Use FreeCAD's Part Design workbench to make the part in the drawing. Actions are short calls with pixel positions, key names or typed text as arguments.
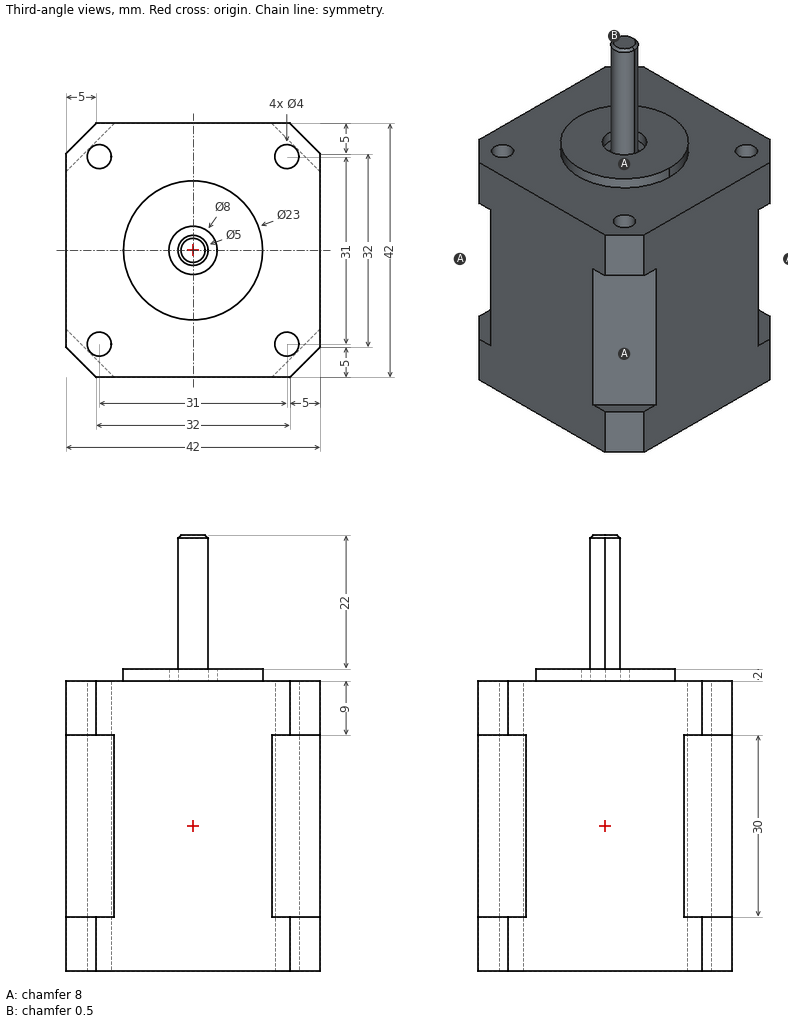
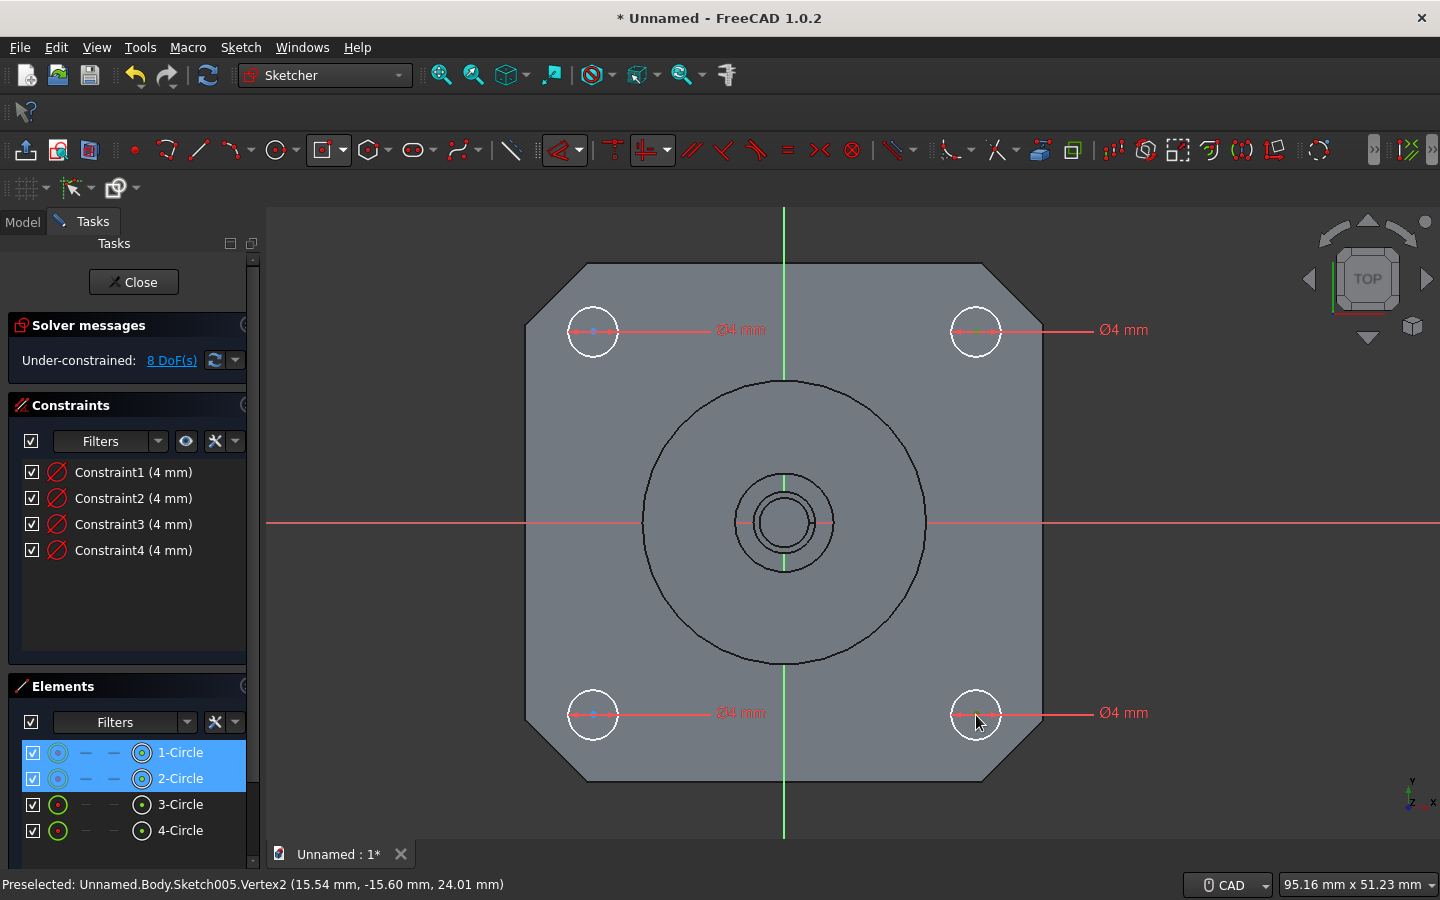
click(364, 523)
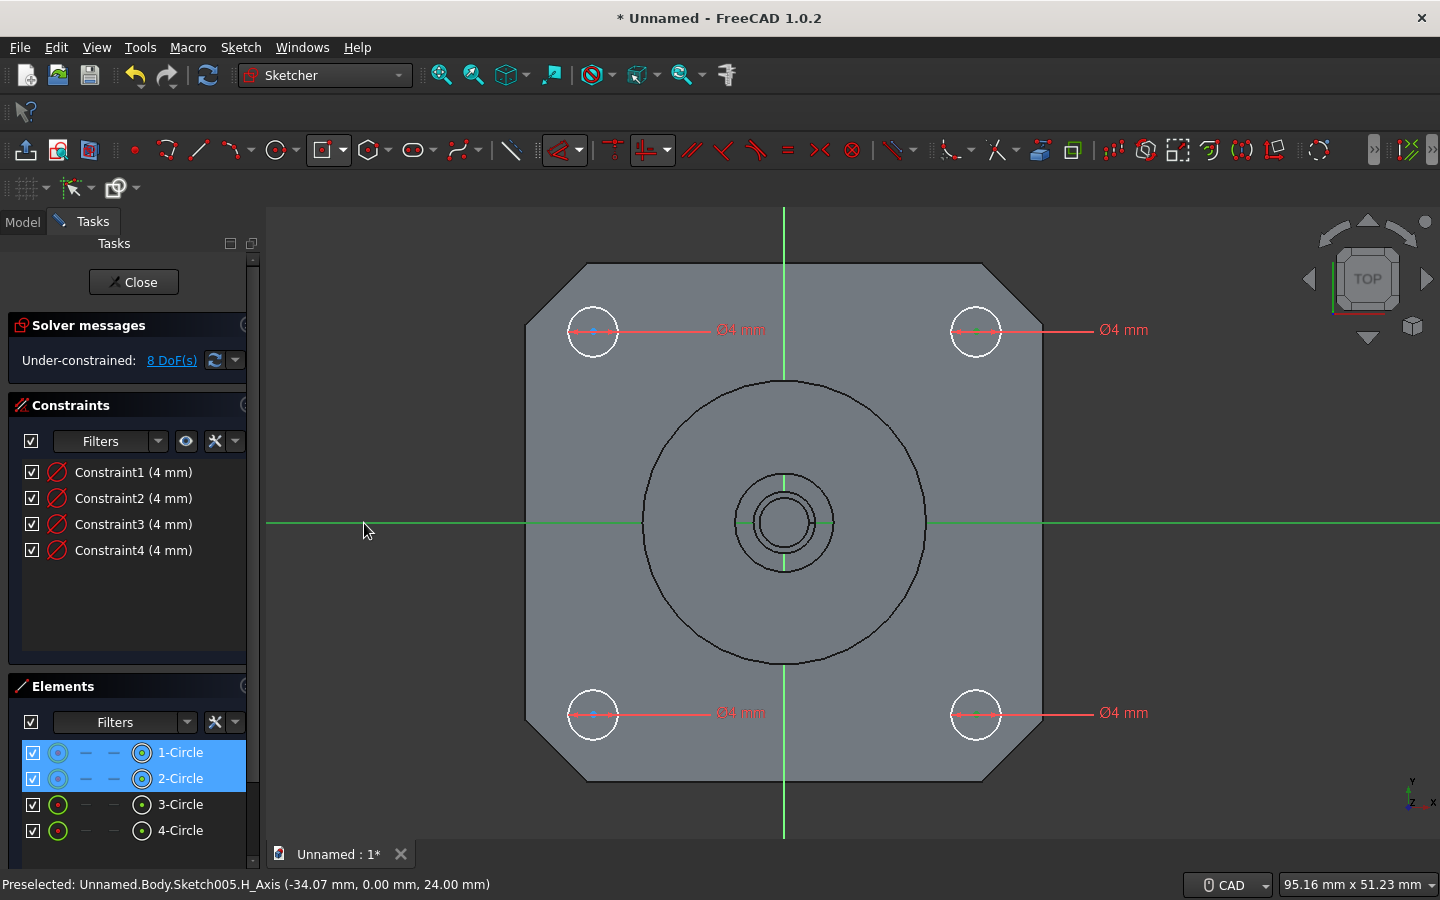
click(820, 150)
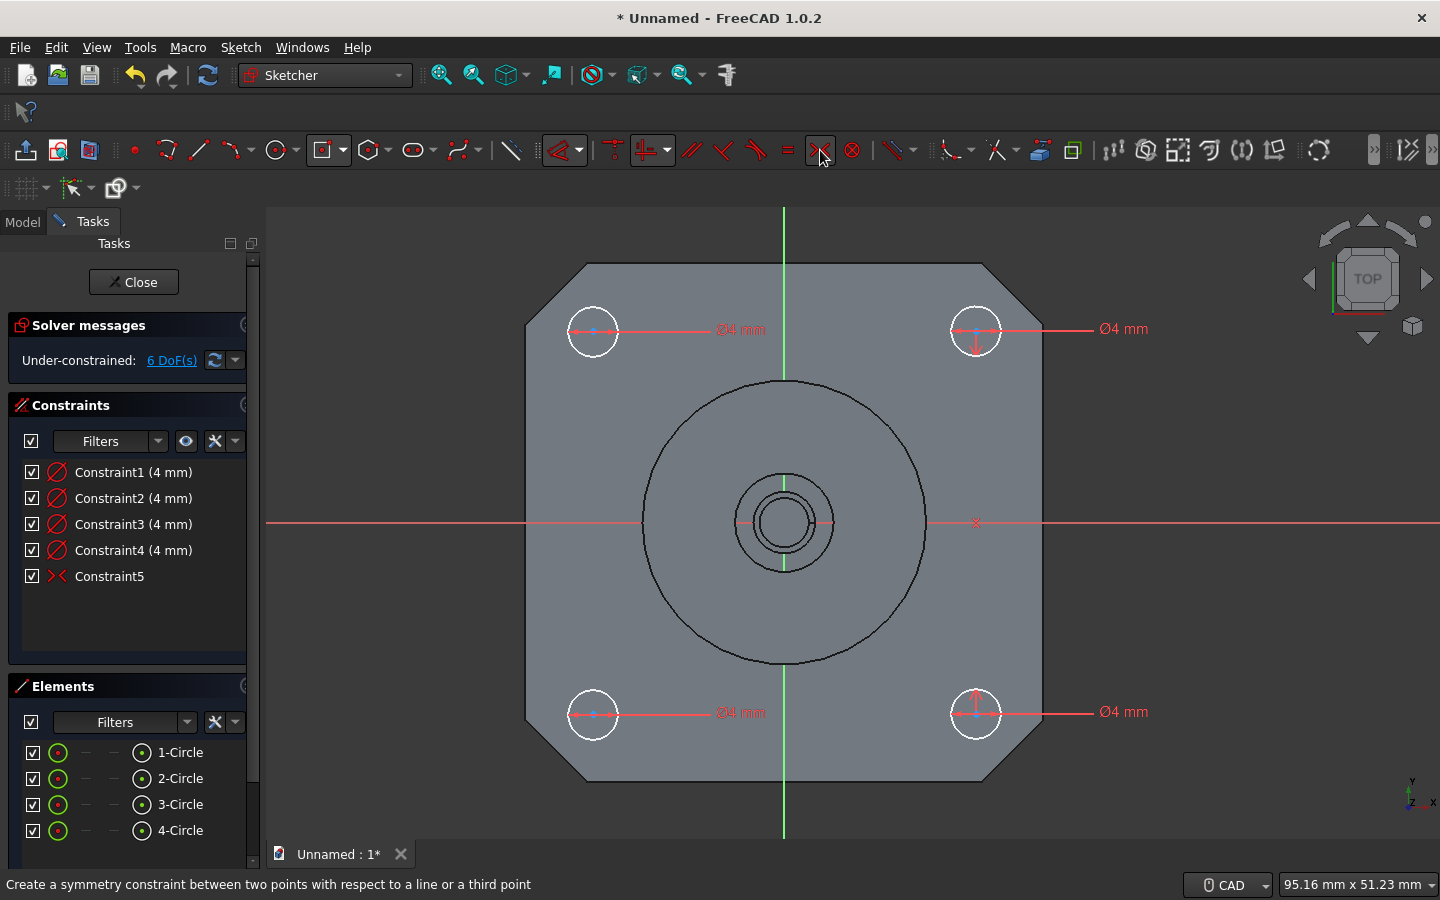
click(976, 714)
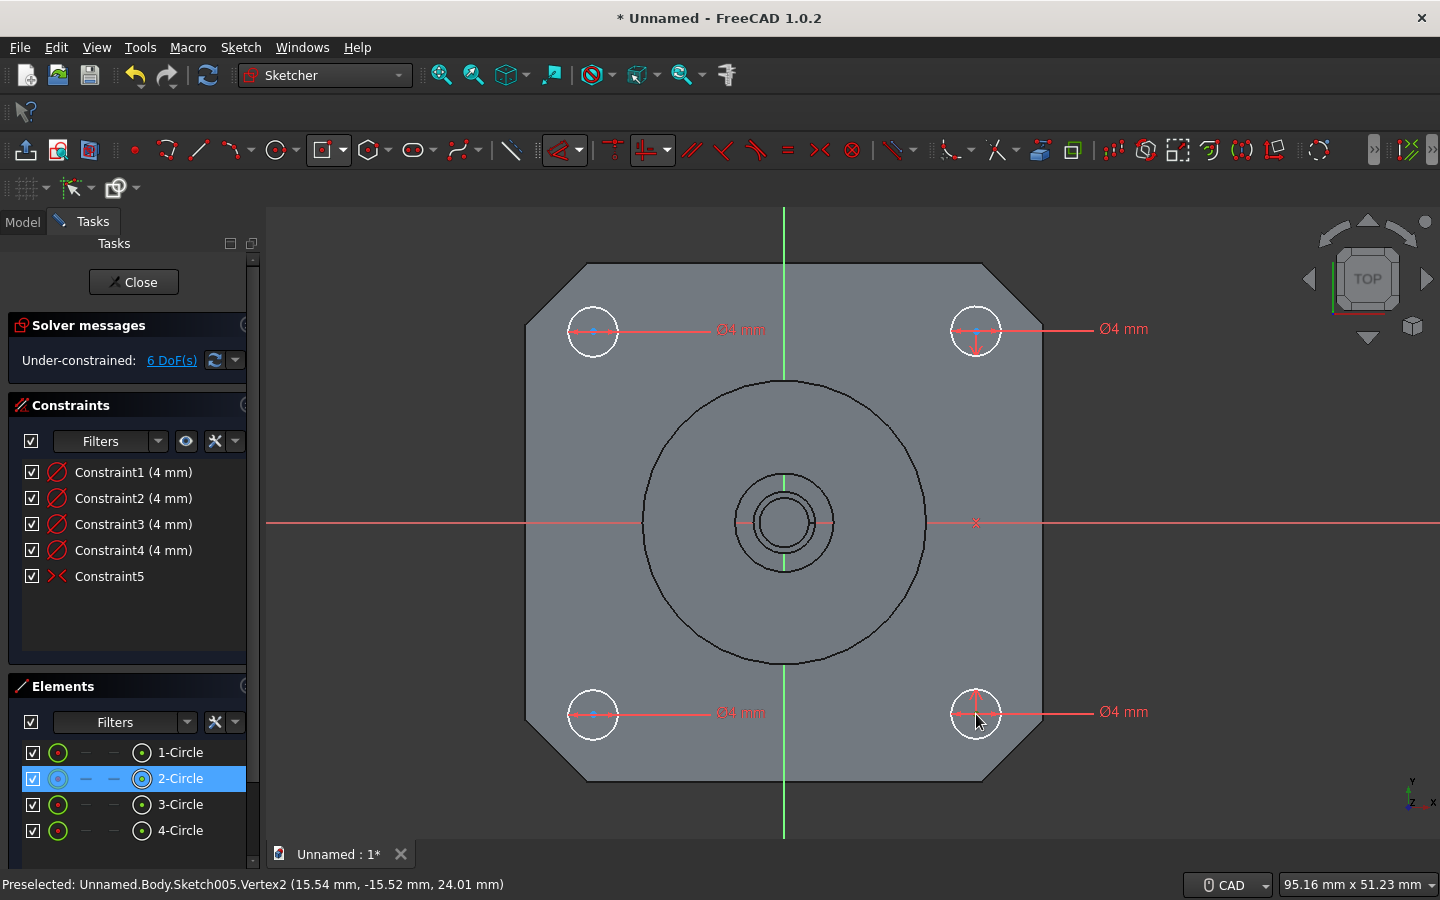
click(593, 715)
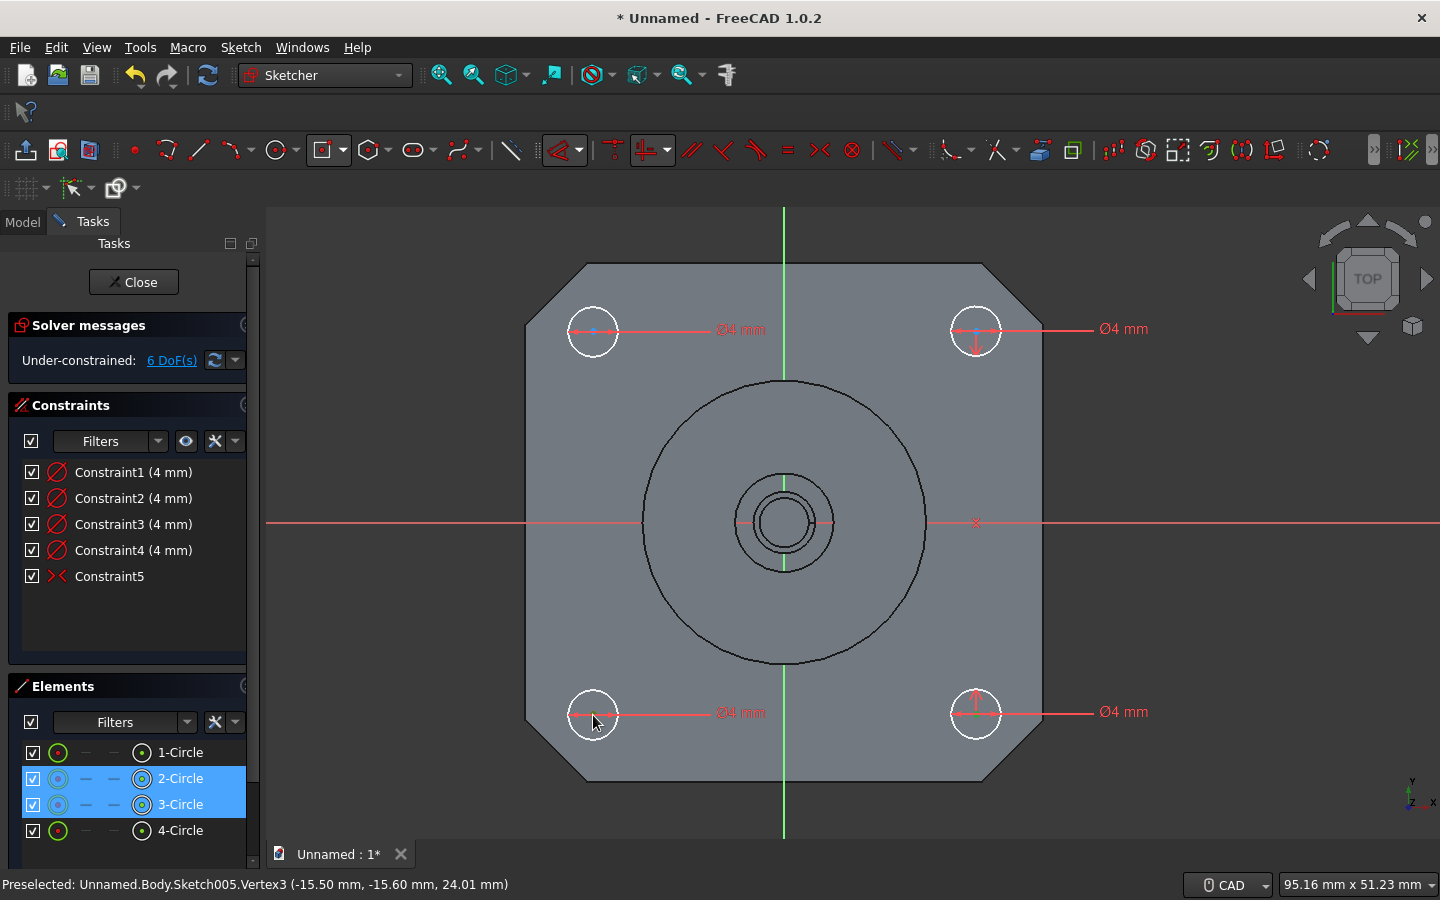
click(784, 770)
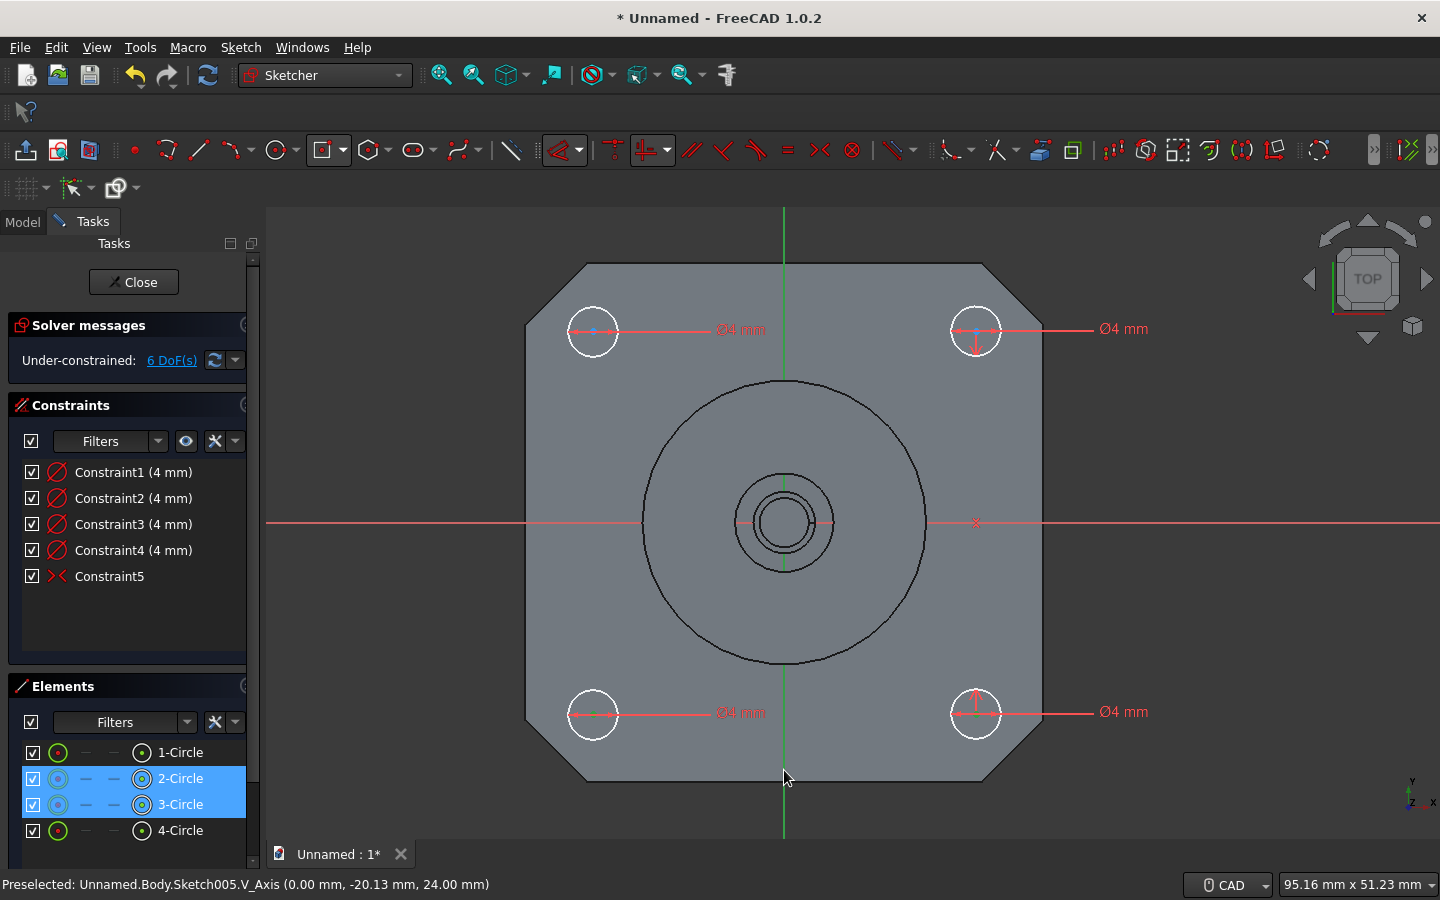
click(820, 150)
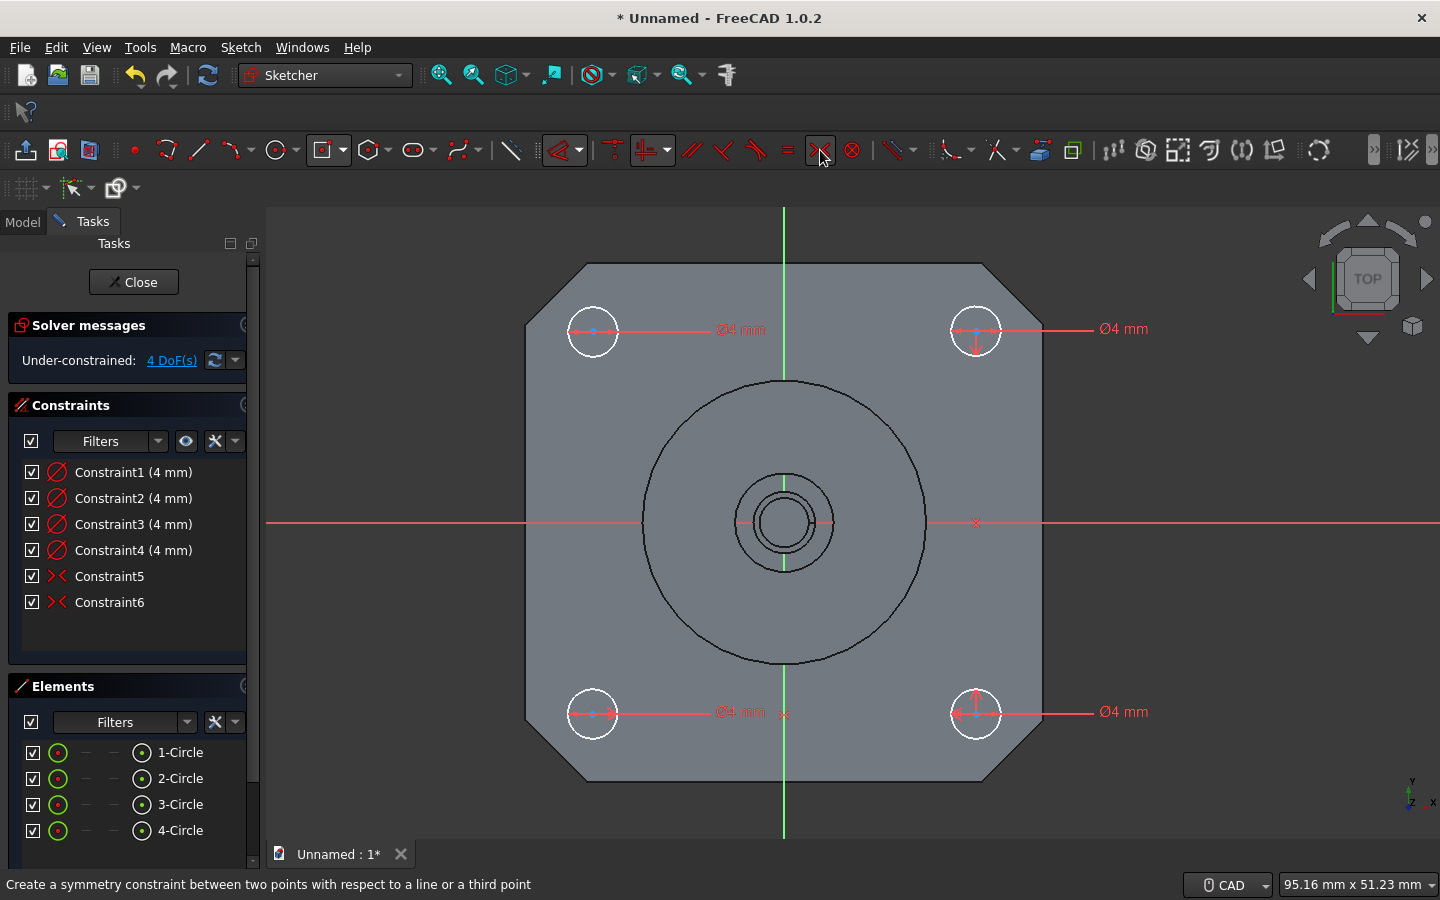
click(976, 331)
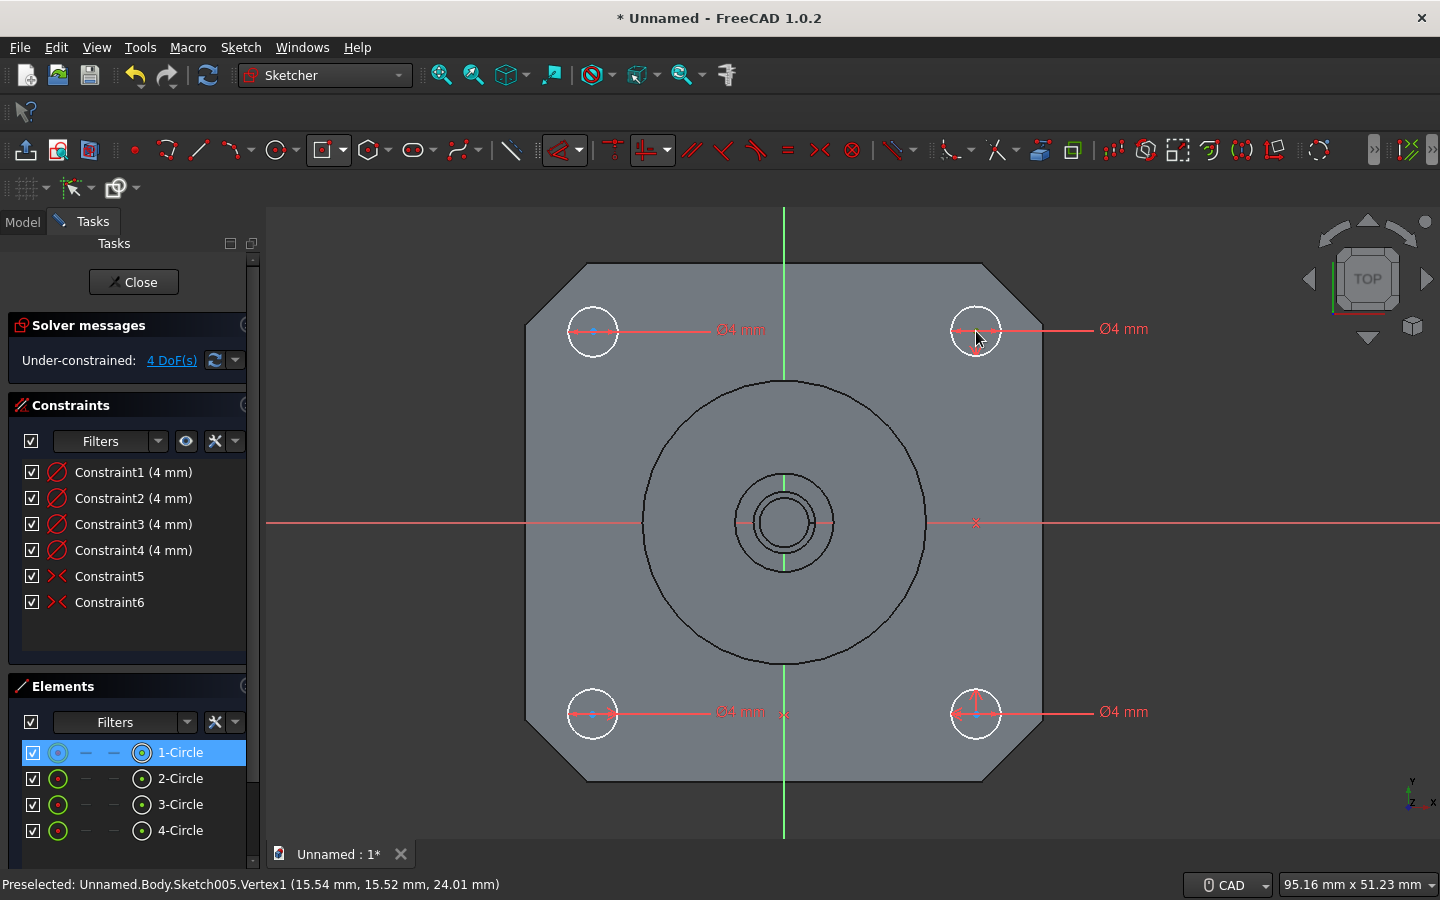
click(593, 332)